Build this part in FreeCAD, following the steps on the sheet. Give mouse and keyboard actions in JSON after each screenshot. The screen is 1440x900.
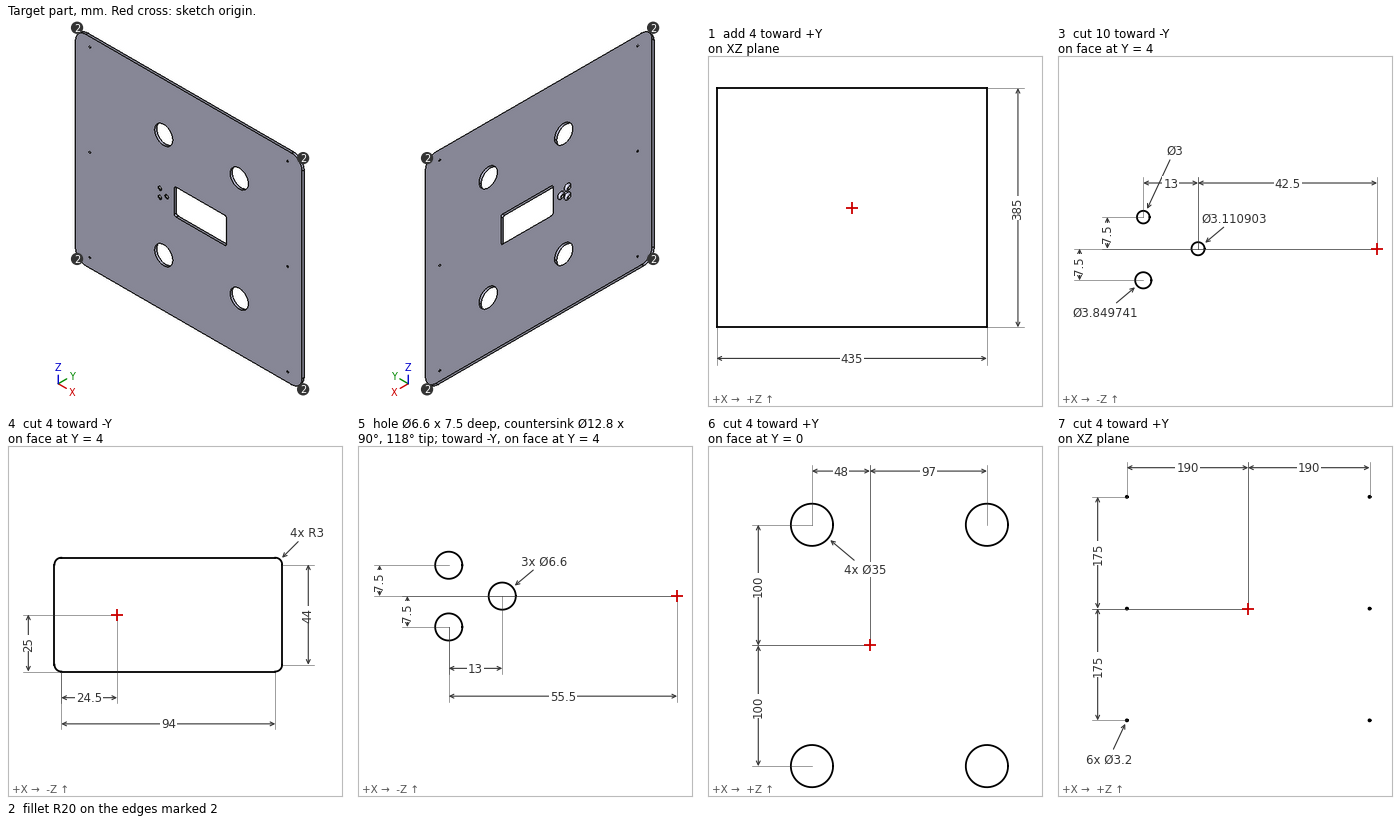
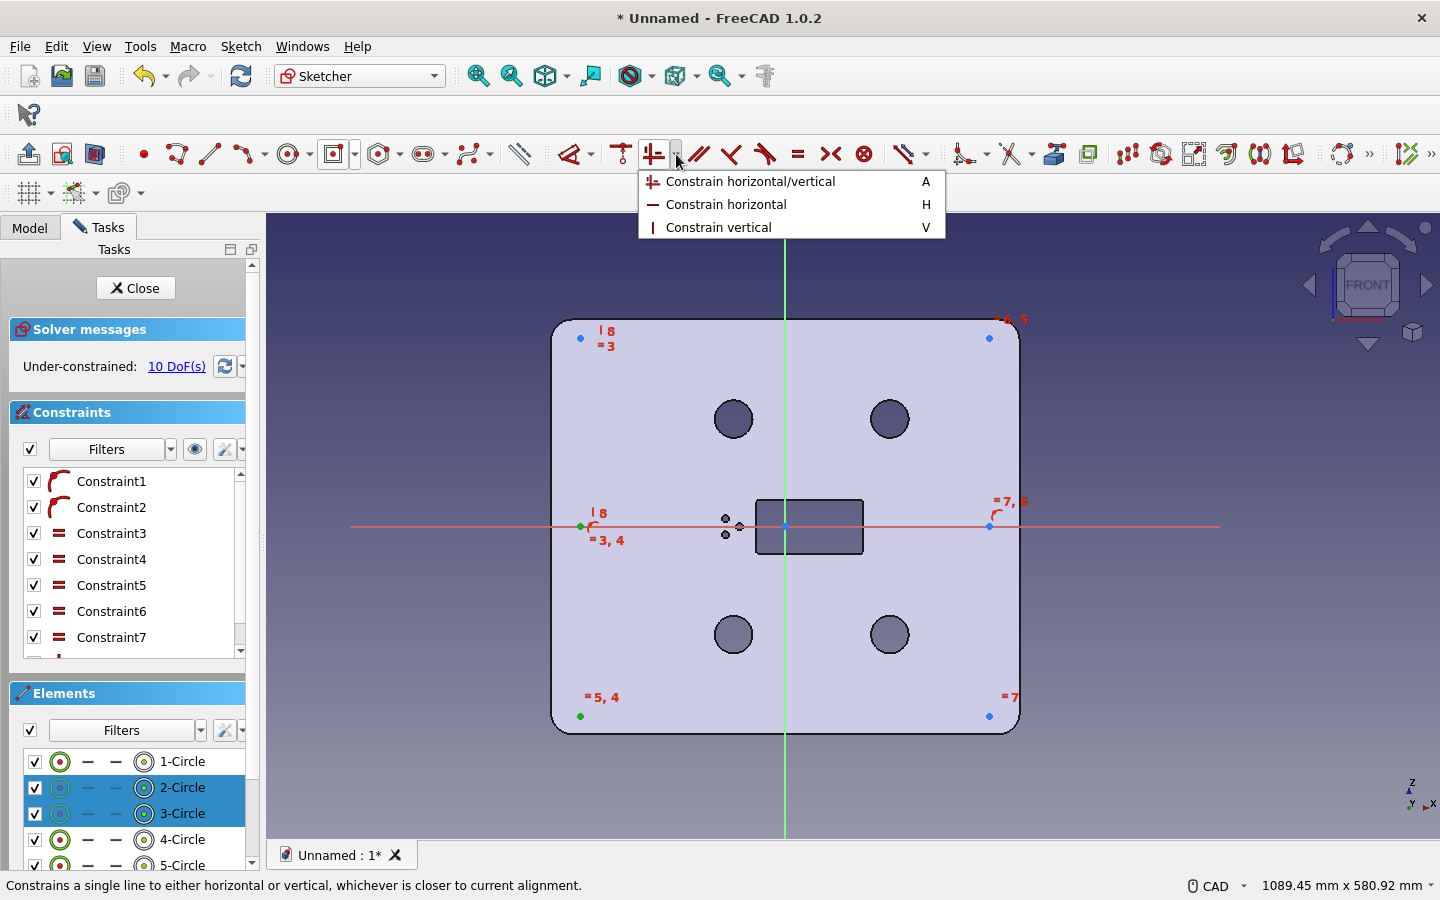
{"action": "left_click", "coordinate": [792, 228]}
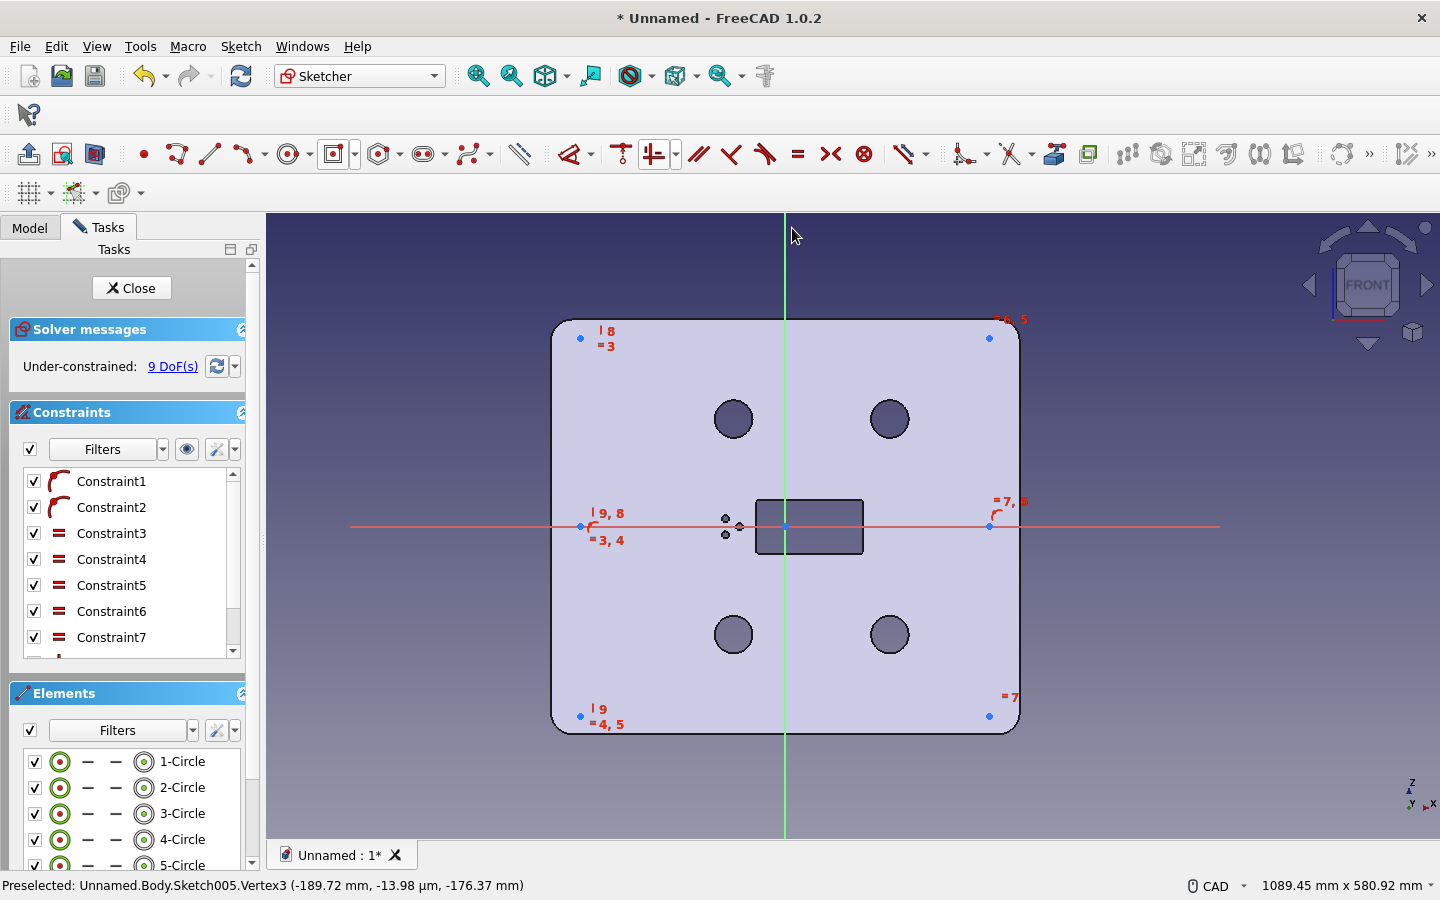
{"action": "left_click", "coordinate": [581, 339]}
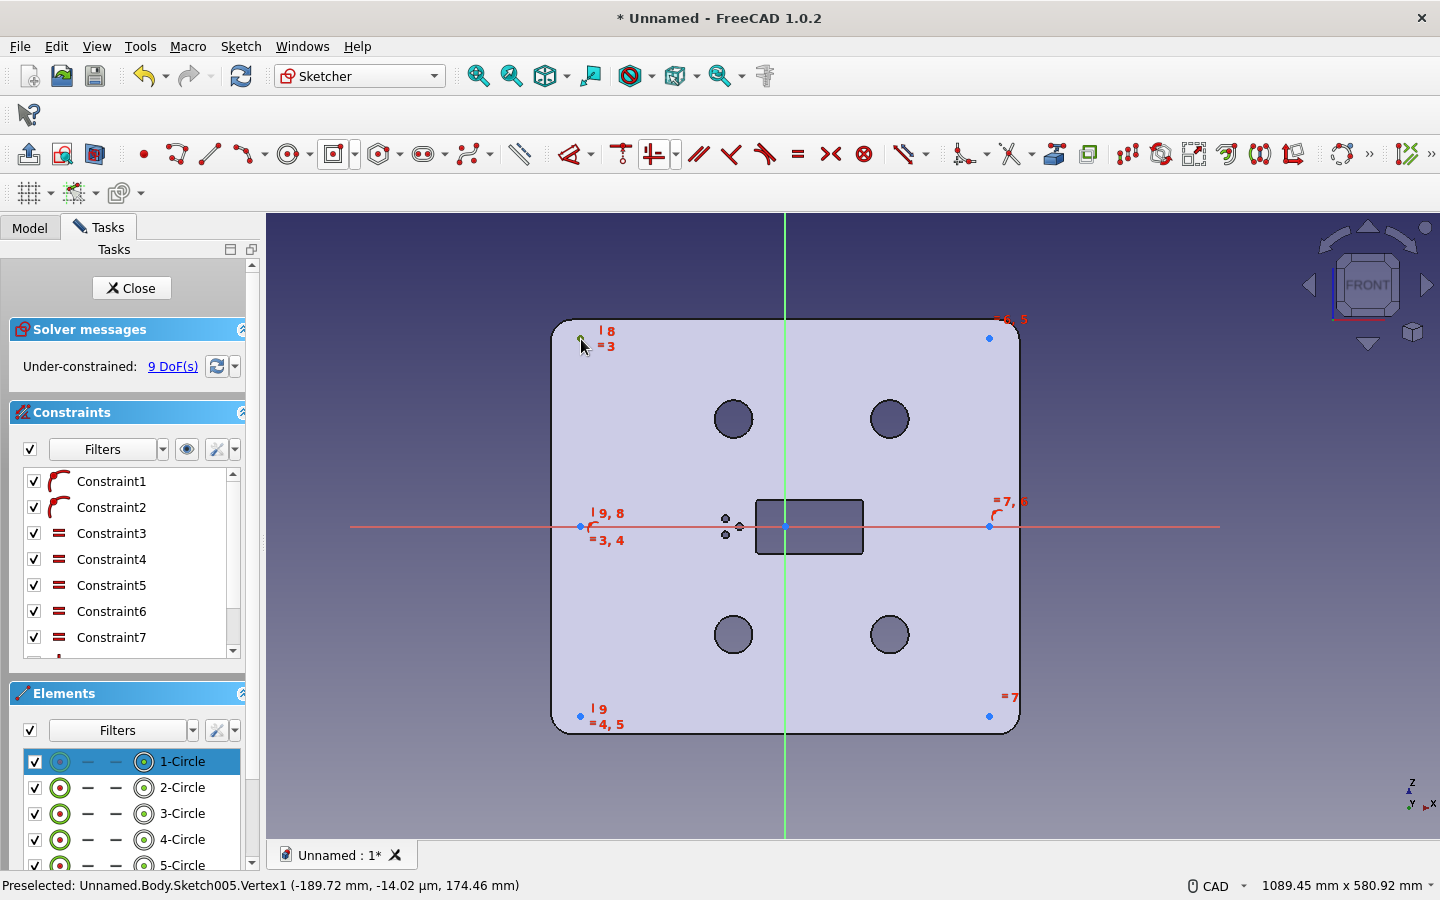
{"action": "left_click", "coordinate": [990, 339]}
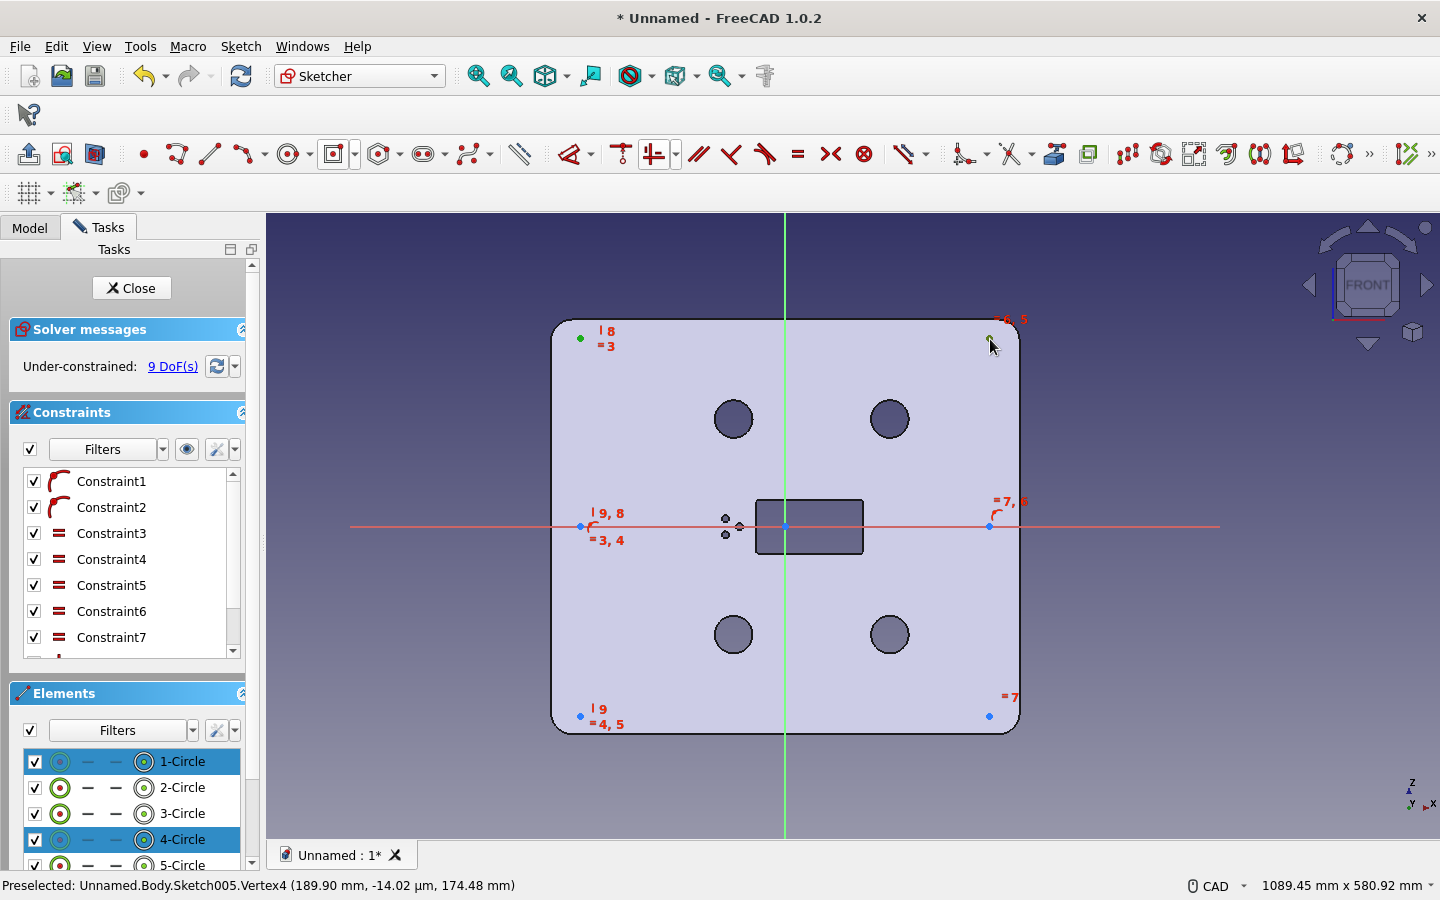
{"action": "key", "text": "h"}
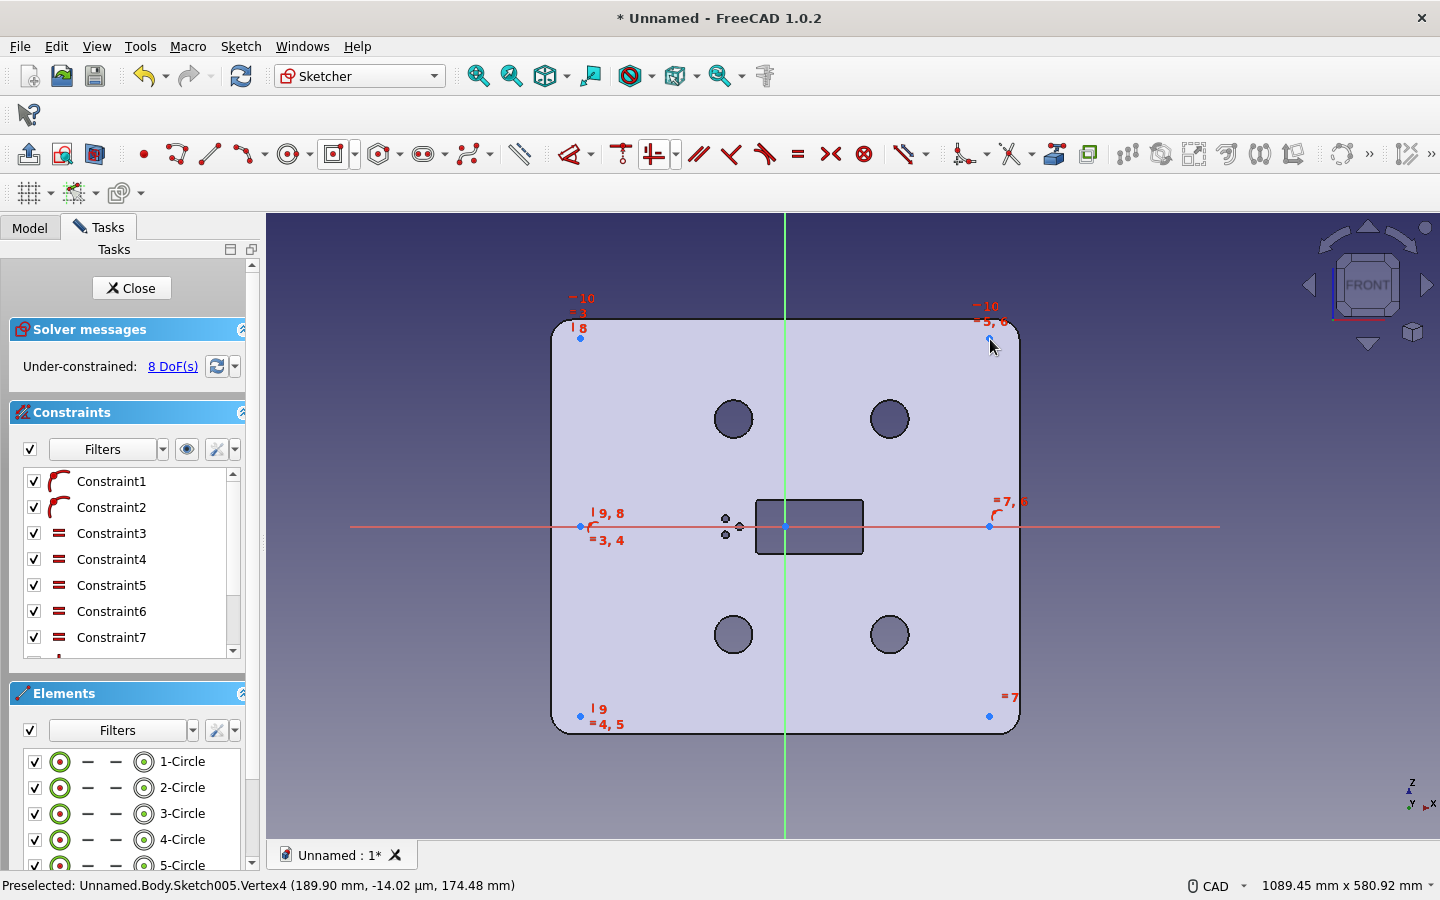
{"action": "left_click", "coordinate": [990, 339]}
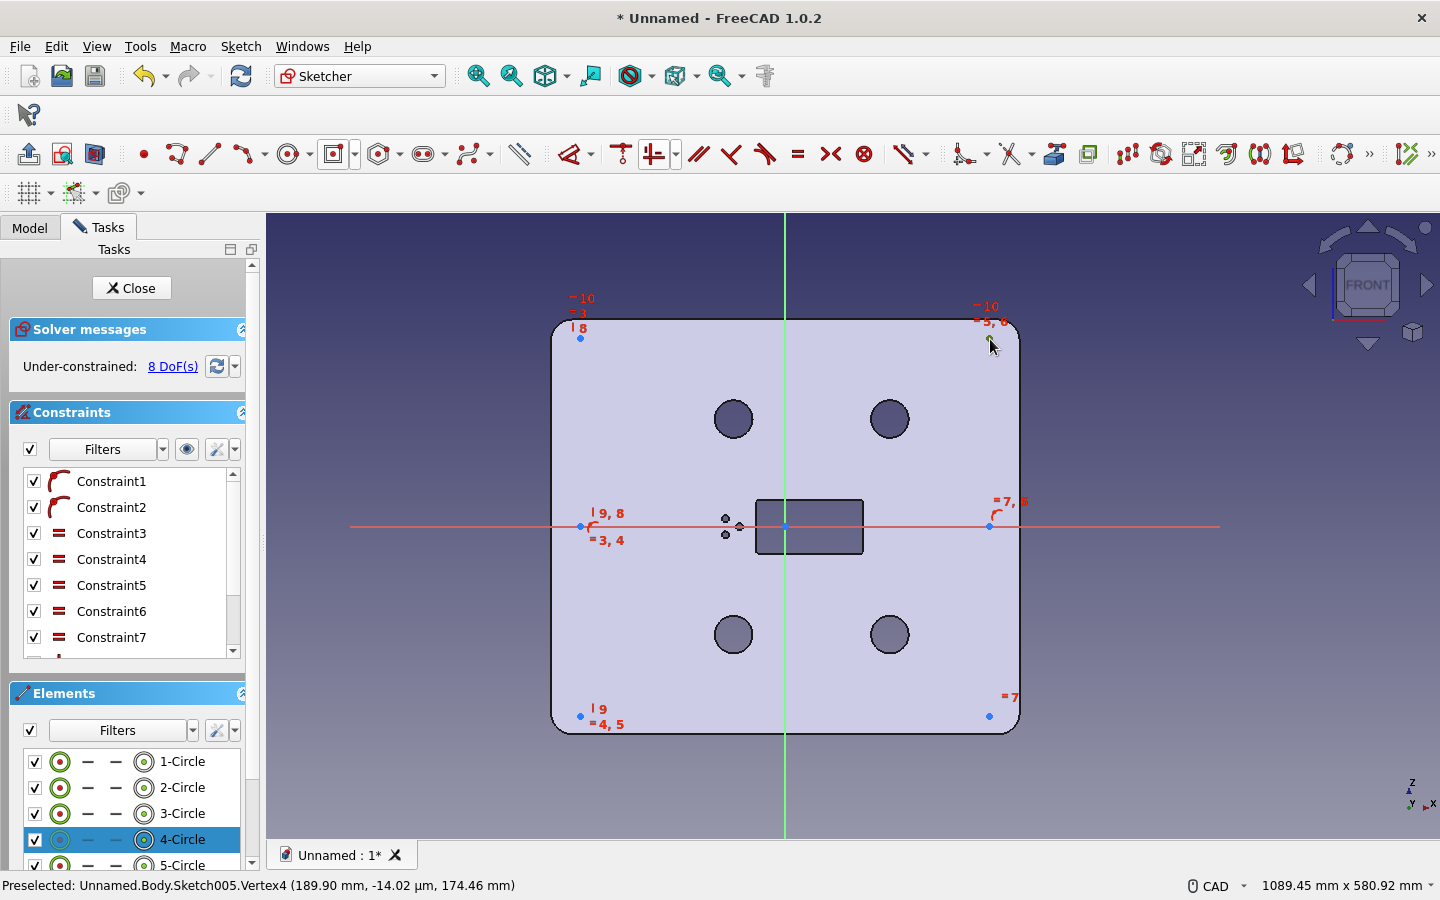
{"action": "left_click", "coordinate": [990, 527]}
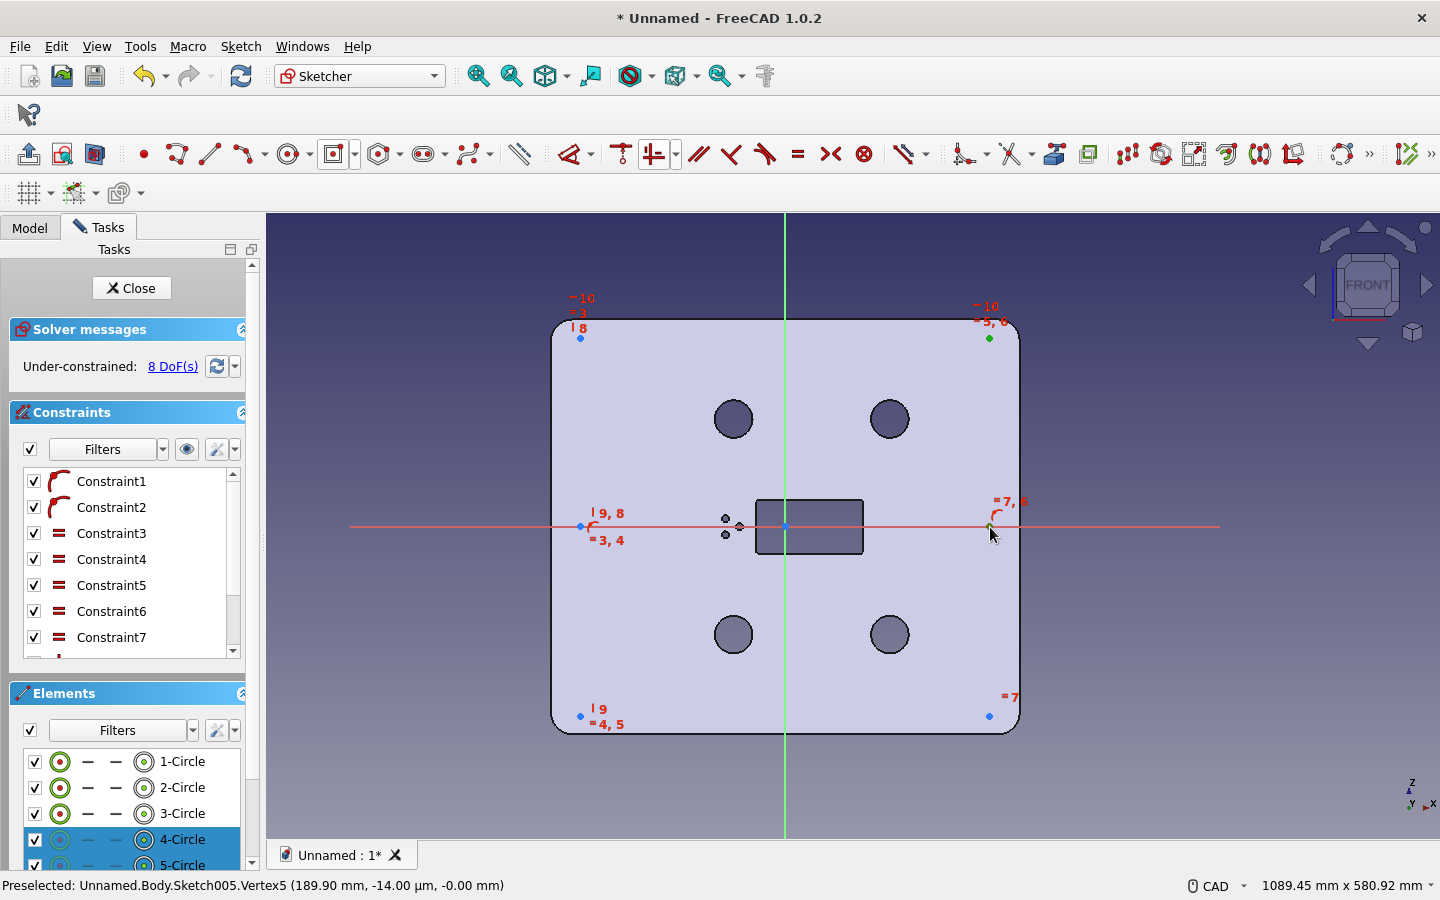
{"action": "key", "text": "v"}